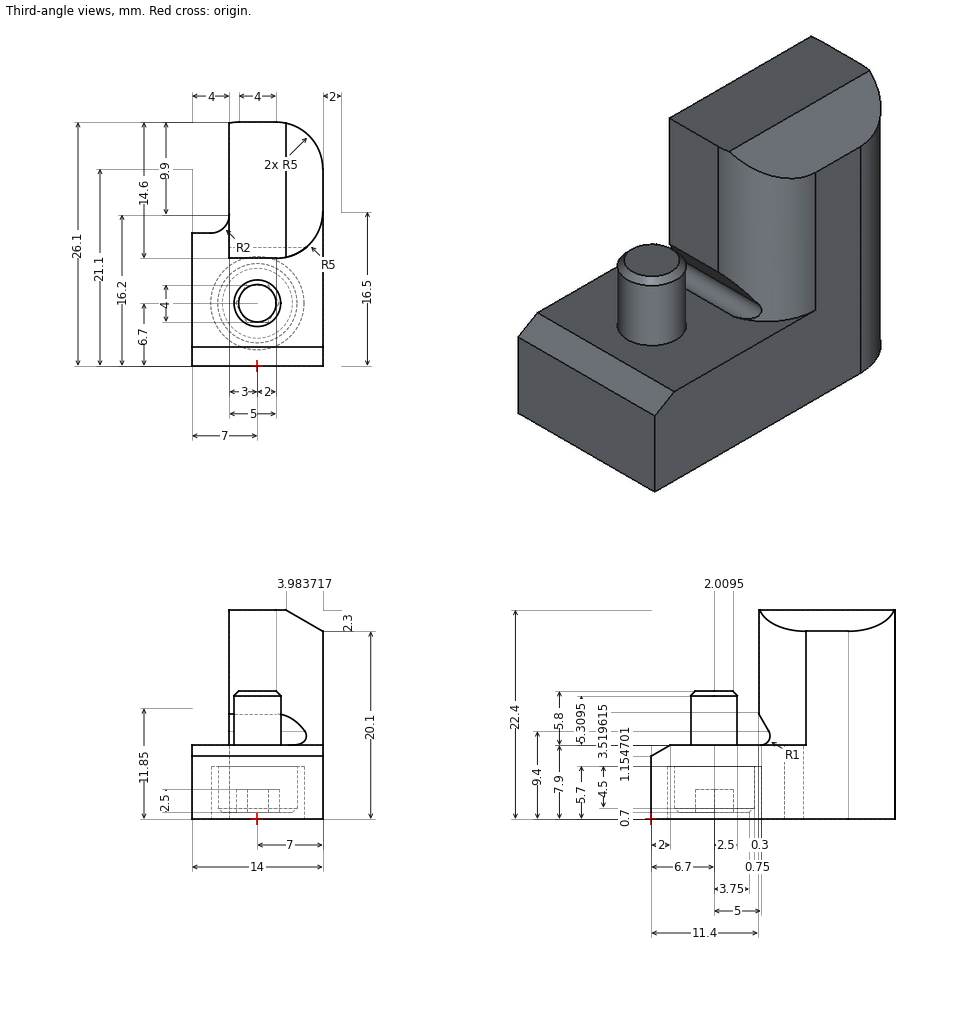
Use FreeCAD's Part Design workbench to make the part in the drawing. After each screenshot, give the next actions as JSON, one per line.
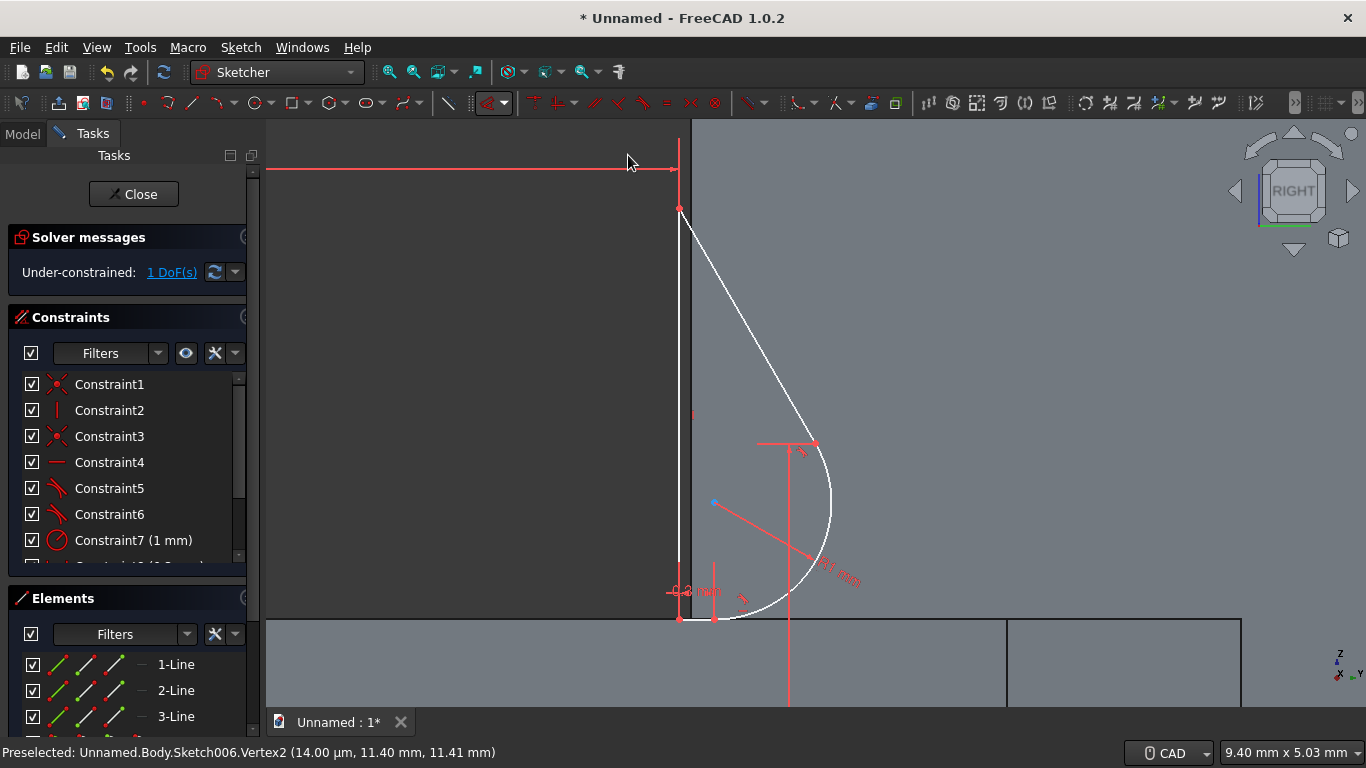
{"action": "left_click", "coordinate": [679, 332]}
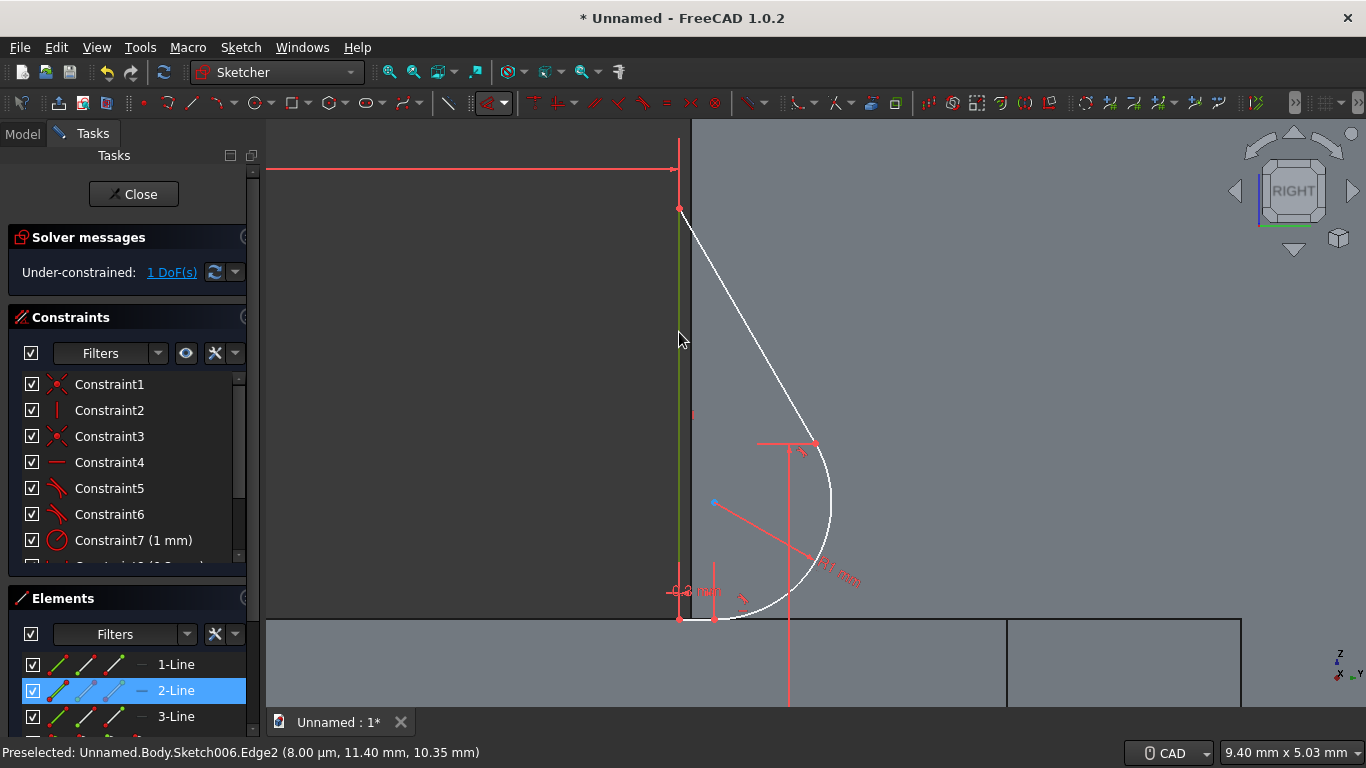
{"action": "key", "text": "i"}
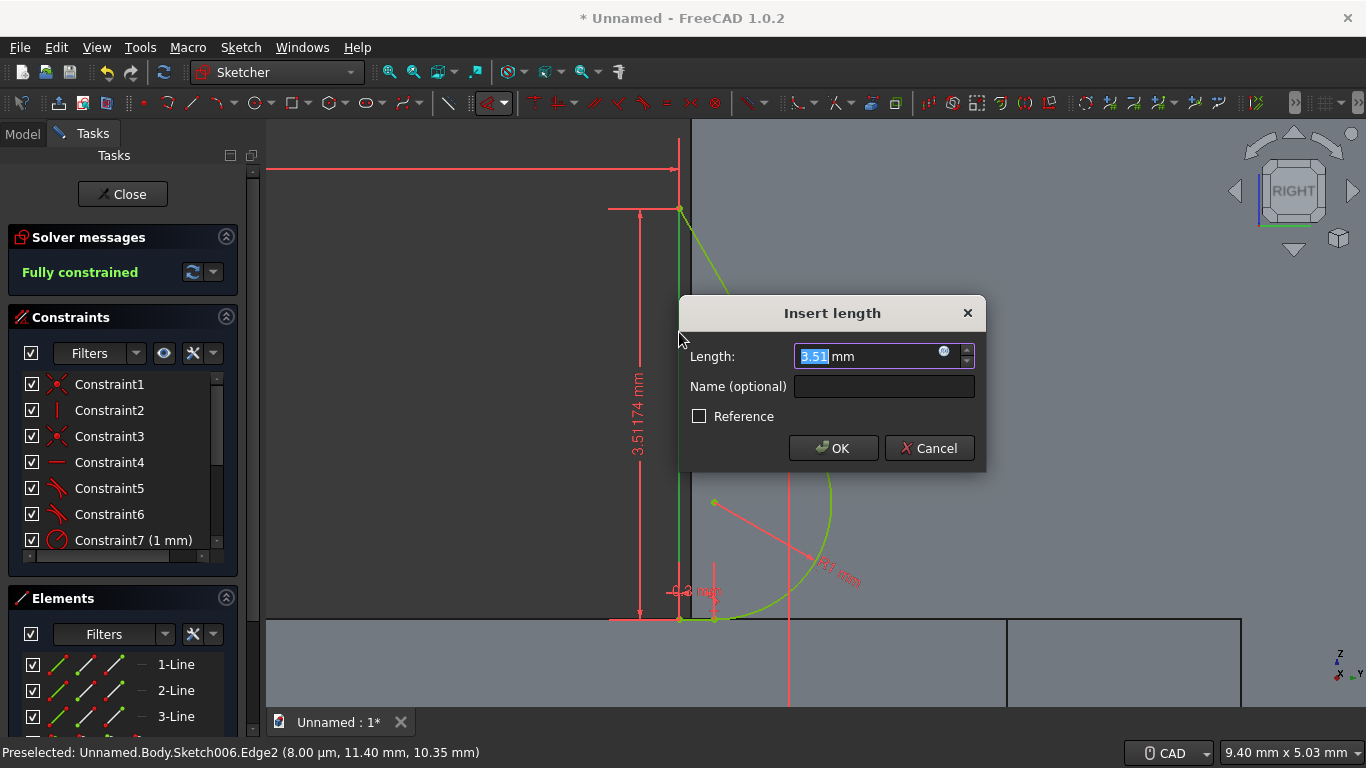
{"action": "type", "text": "3.519615"}
{"action": "key", "text": "Return"}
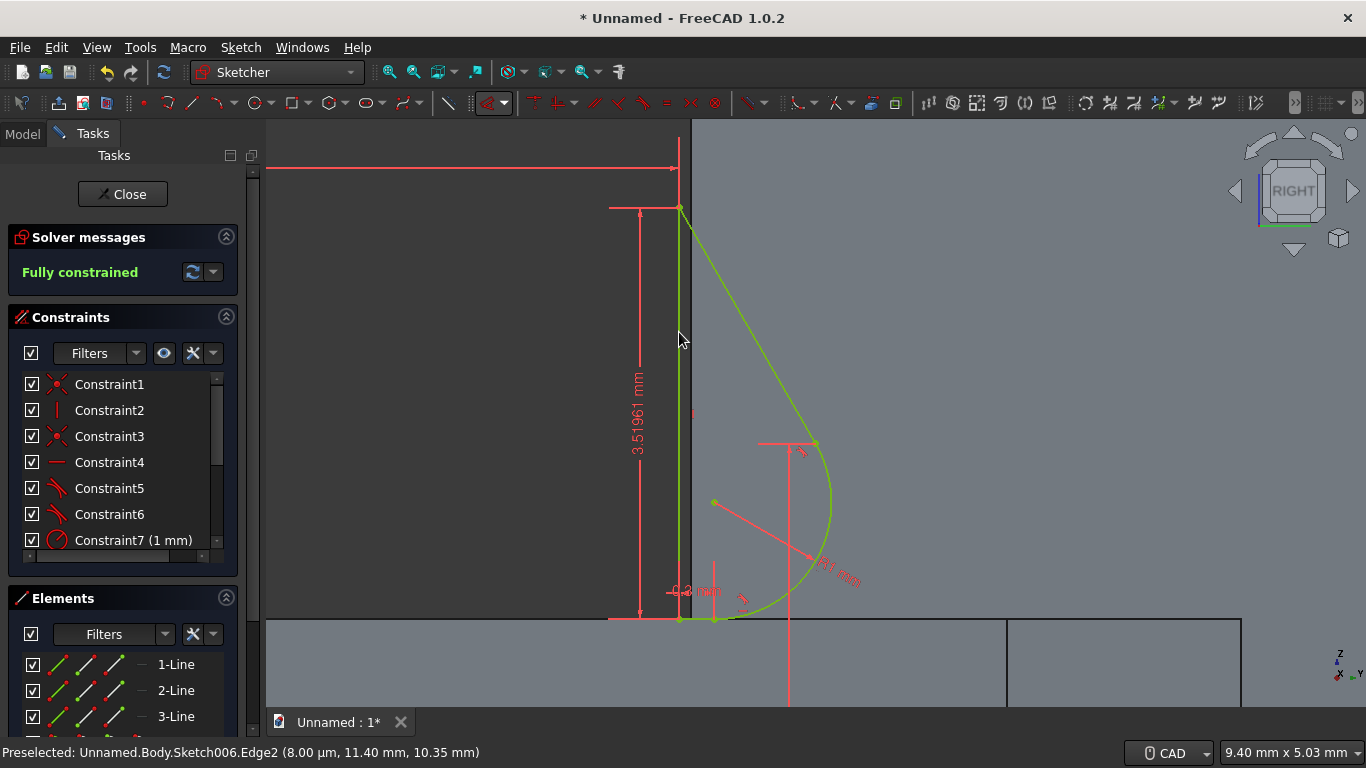
{"action": "left_click", "coordinate": [123, 194]}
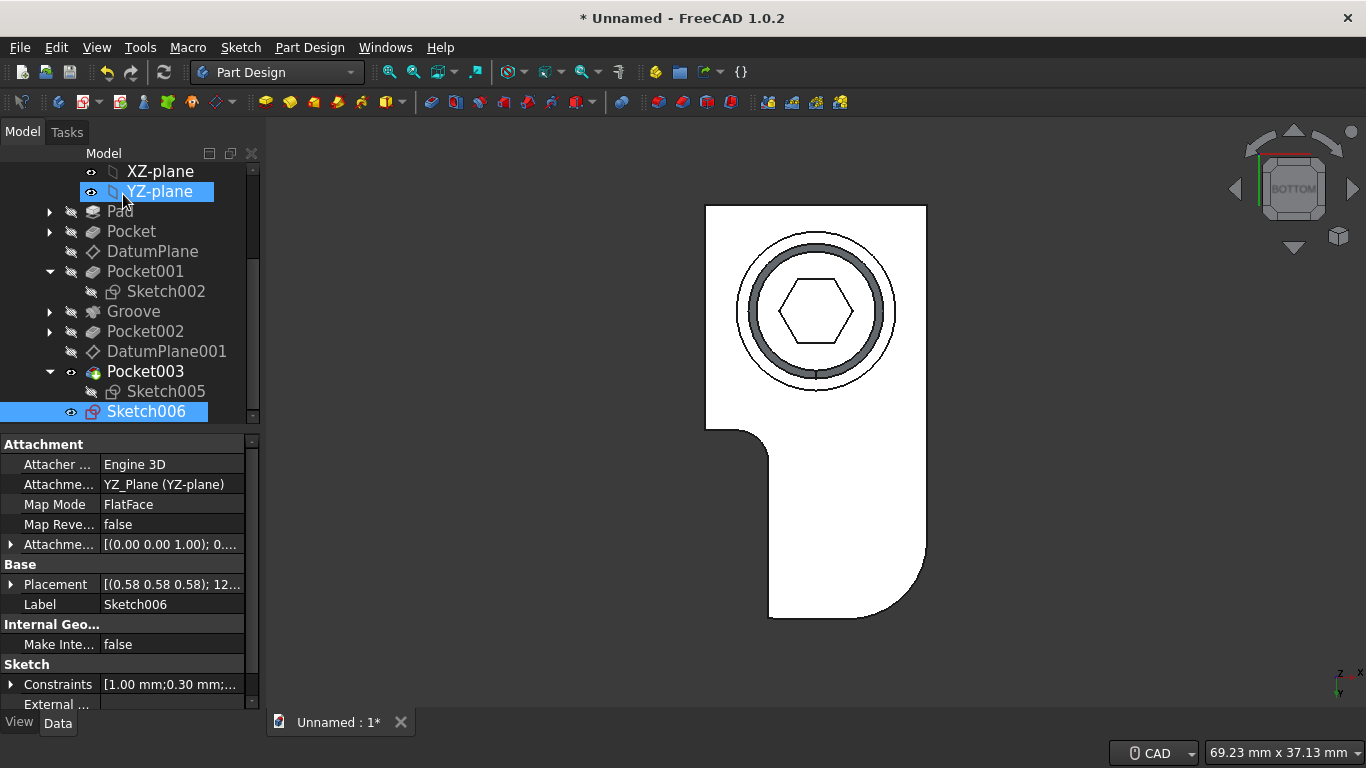
{"action": "left_click", "coordinate": [432, 102]}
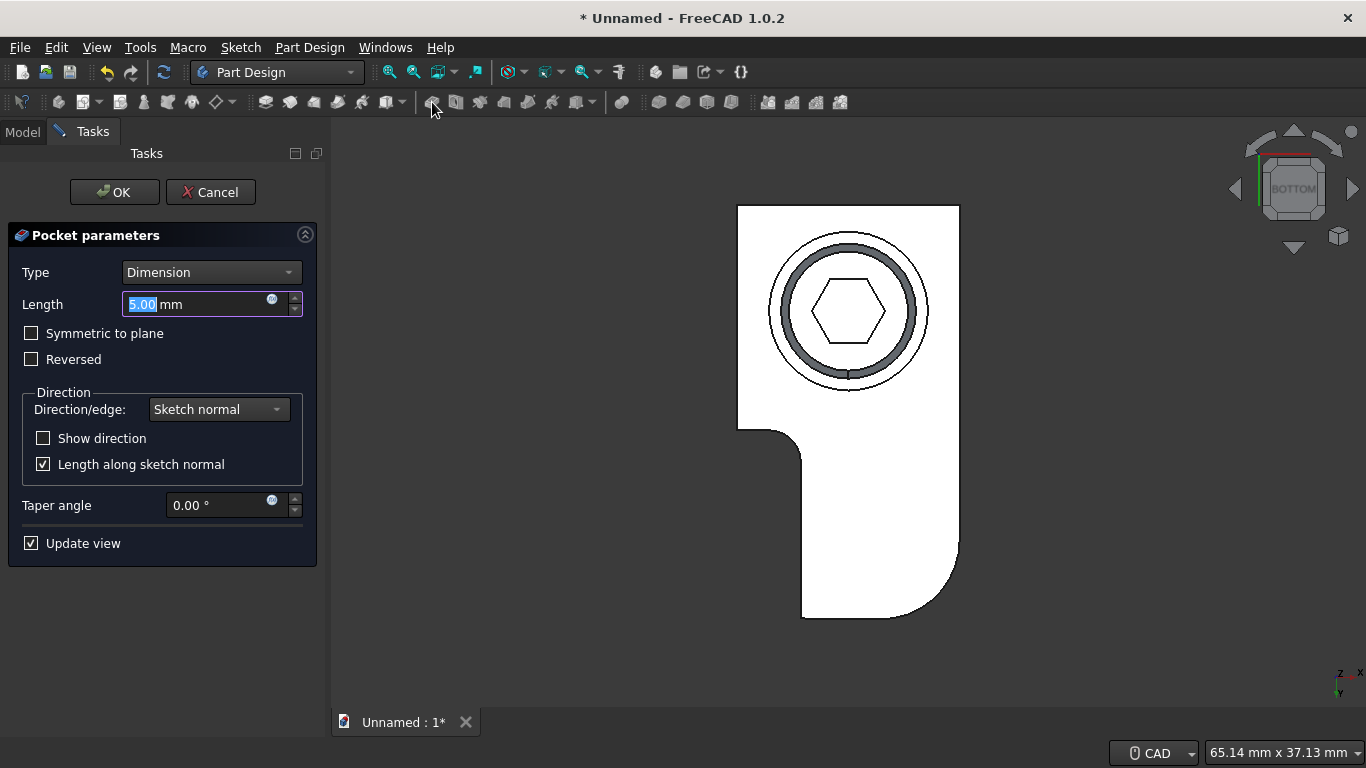
{"action": "type", "text": "14"}
{"action": "key", "text": "Tab"}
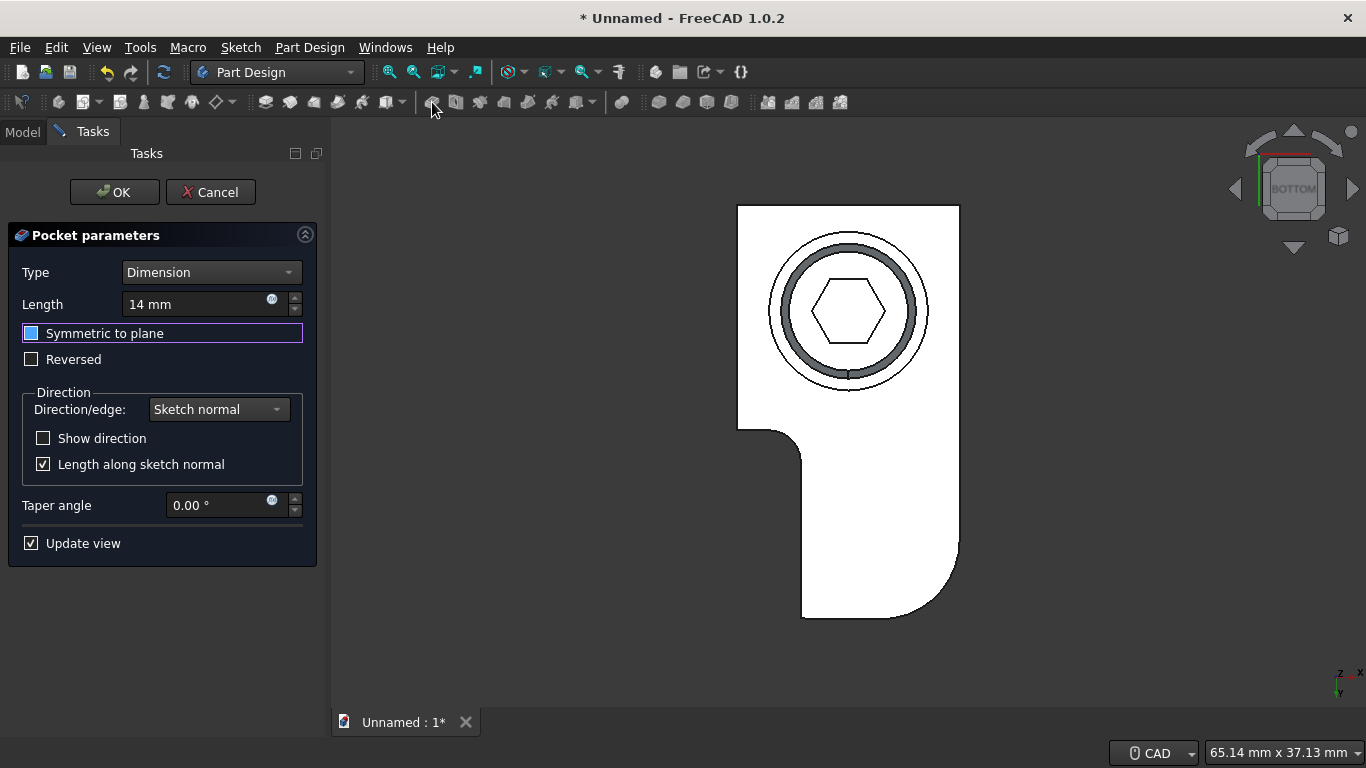
{"action": "left_click", "coordinate": [30, 333]}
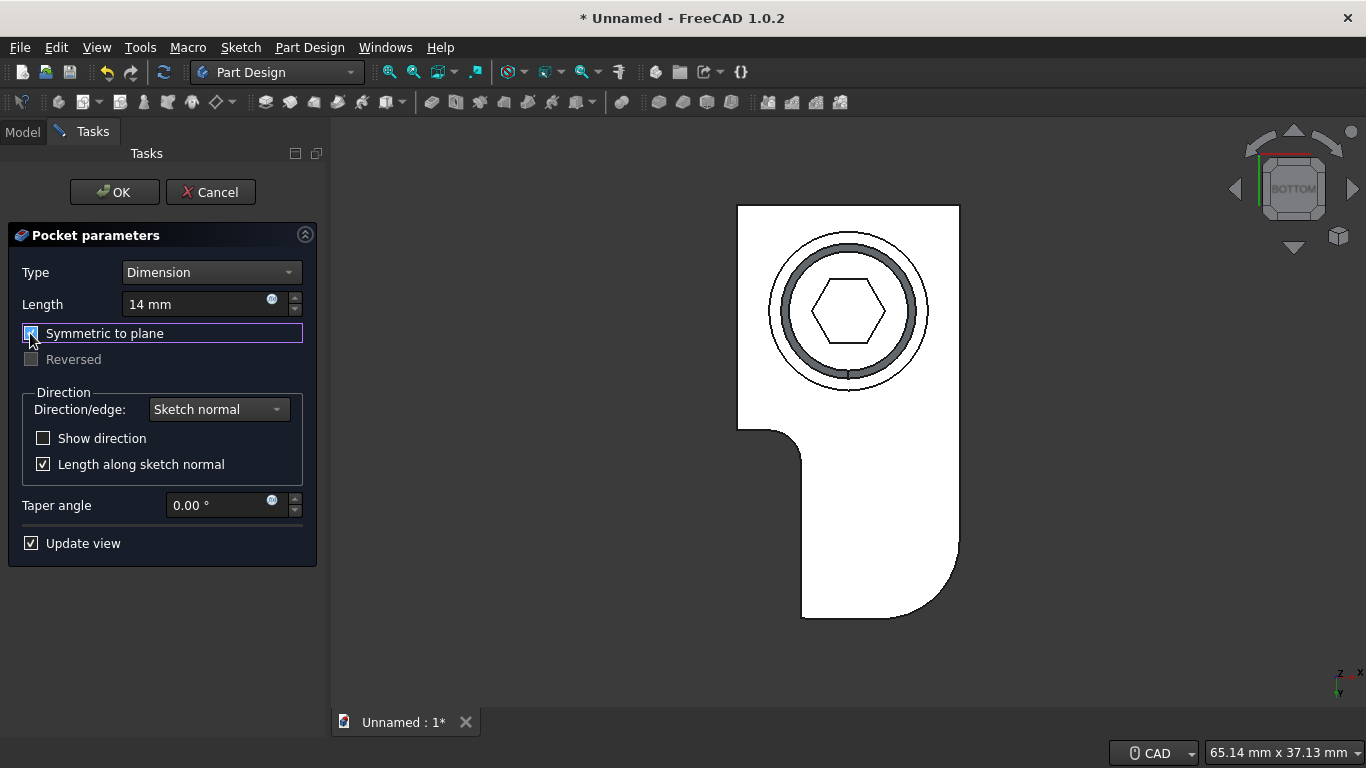
{"action": "left_click", "coordinate": [115, 192]}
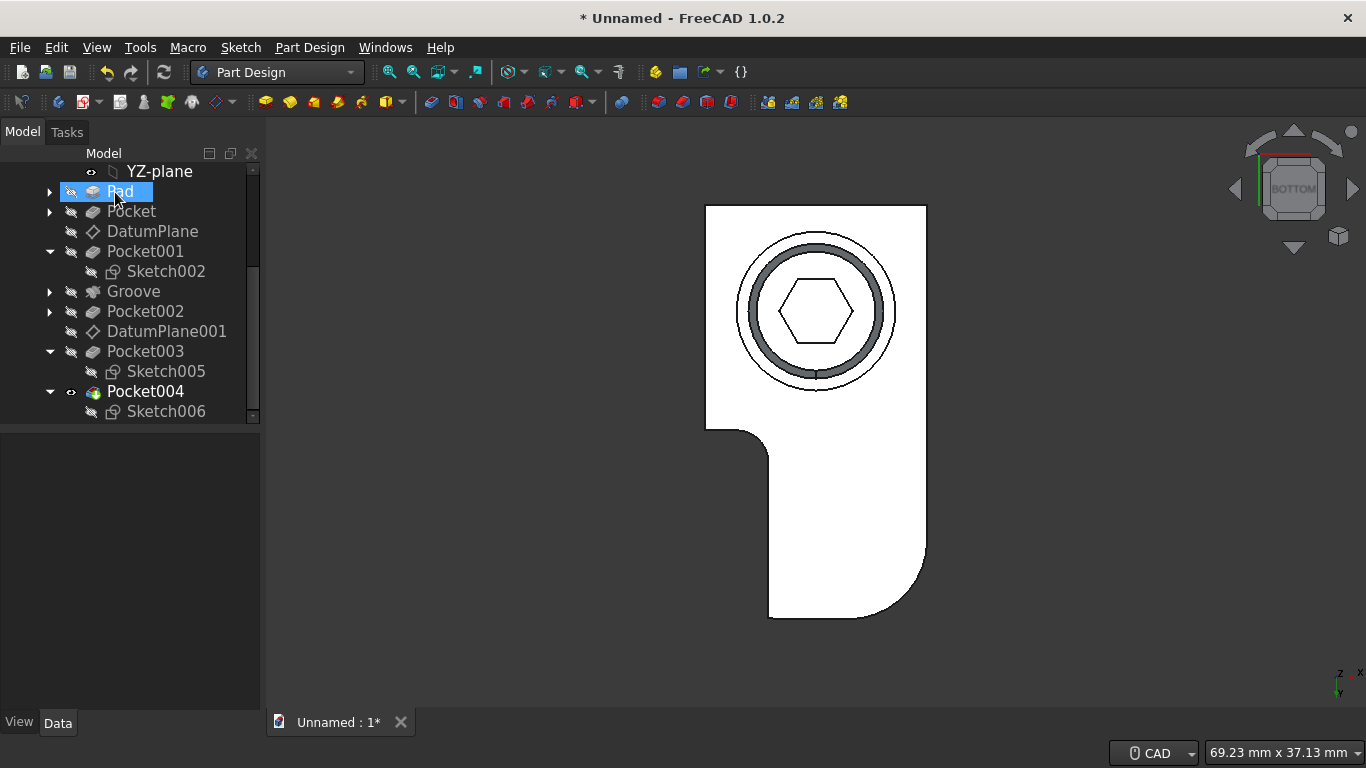
{"action": "key", "text": "0"}